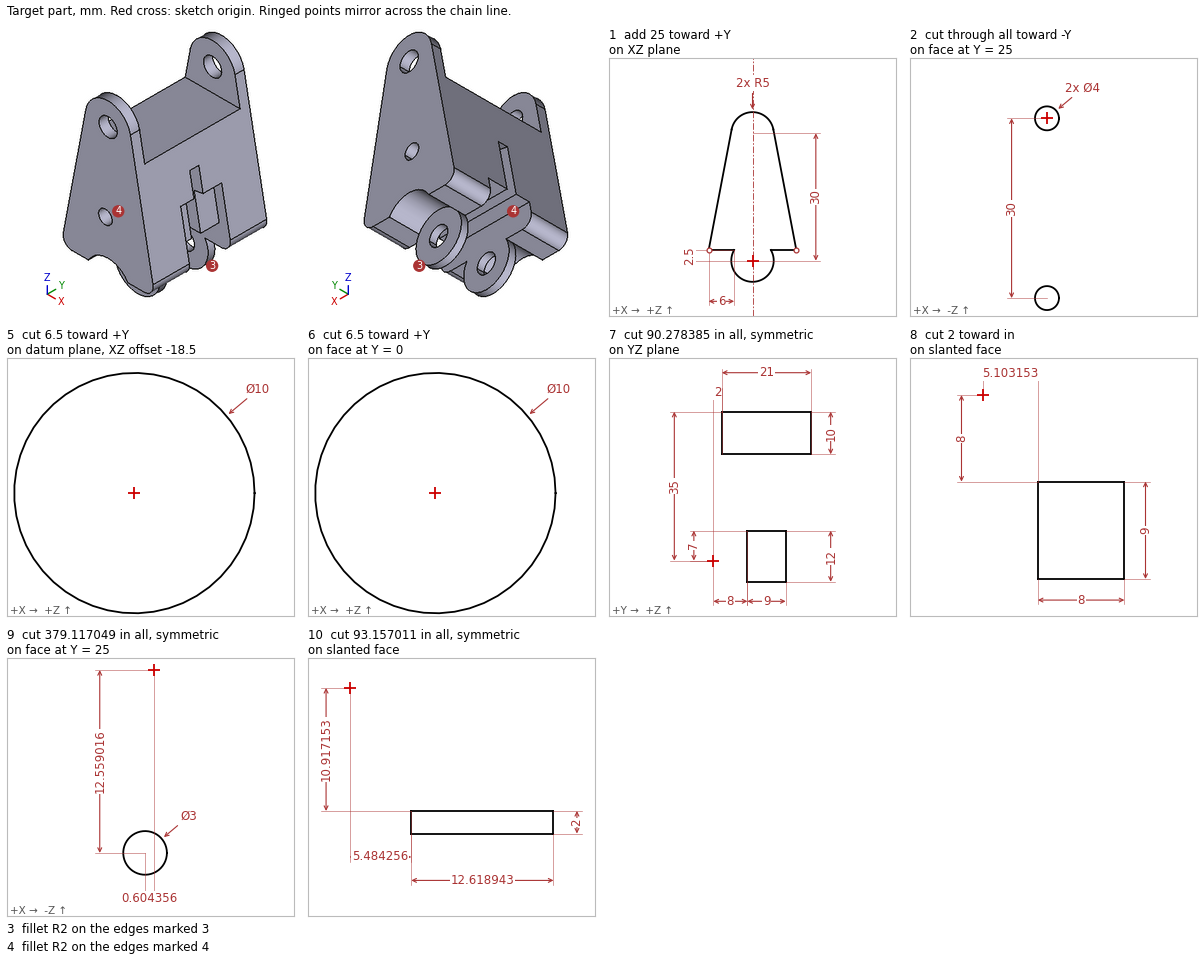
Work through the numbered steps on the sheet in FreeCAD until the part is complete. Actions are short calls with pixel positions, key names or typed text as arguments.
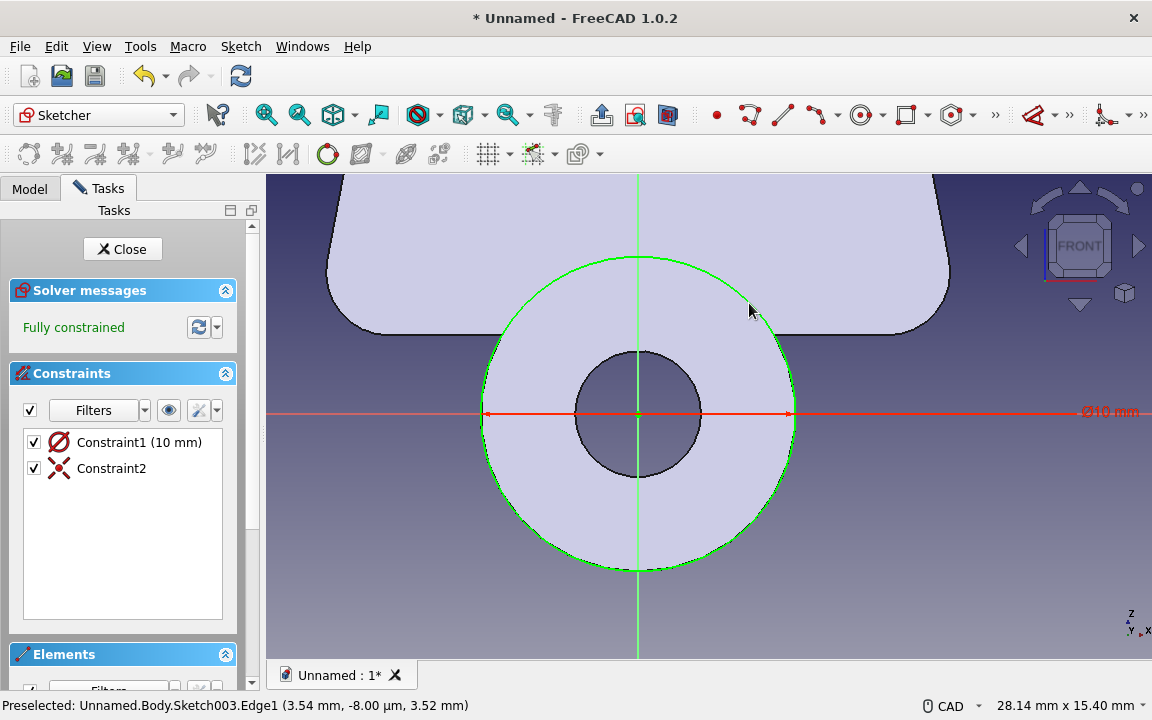
click(123, 249)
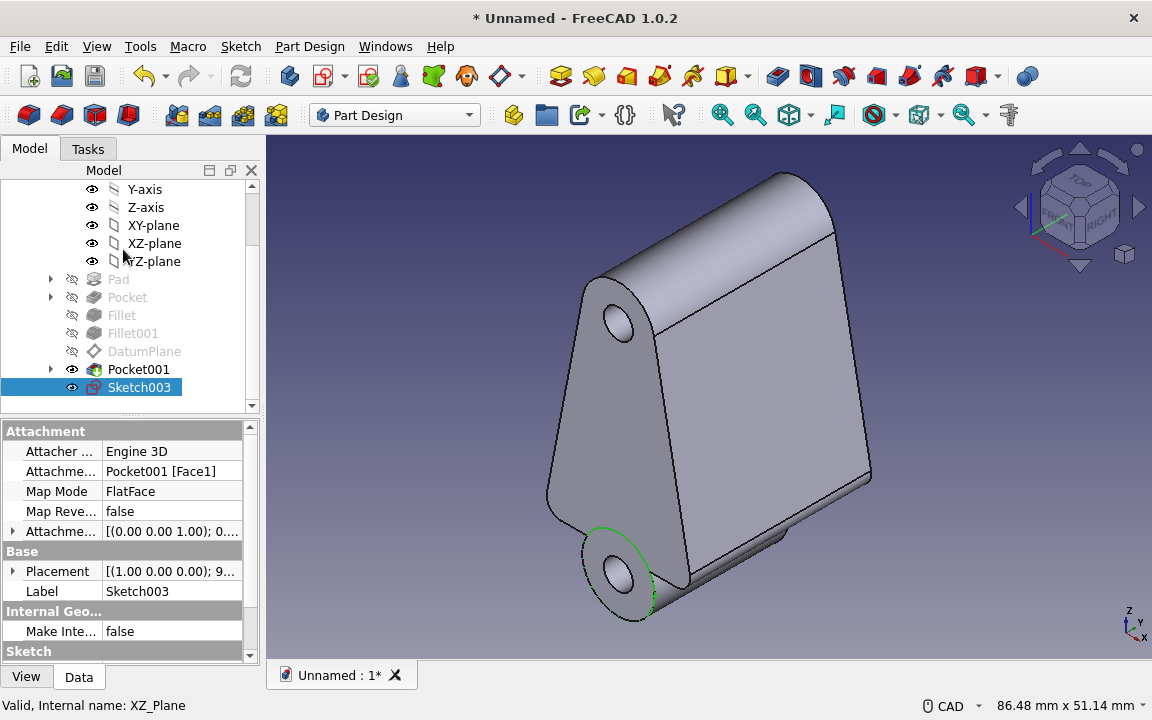
click(778, 76)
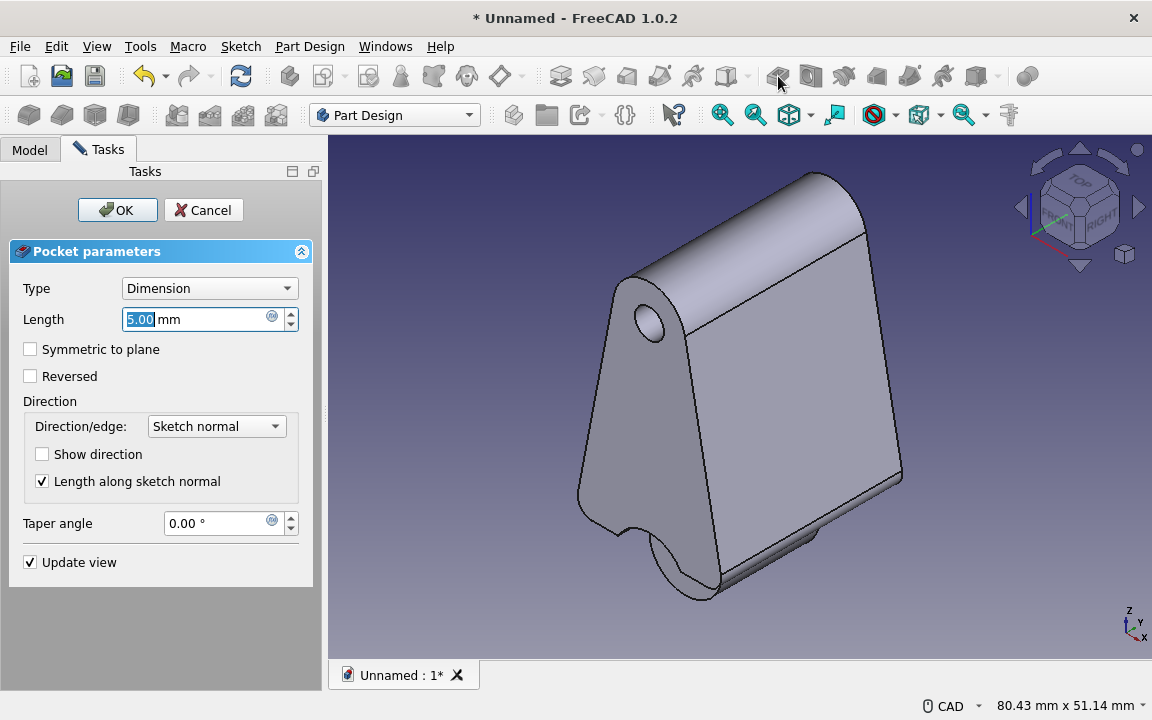
text(6.5)
key(Tab)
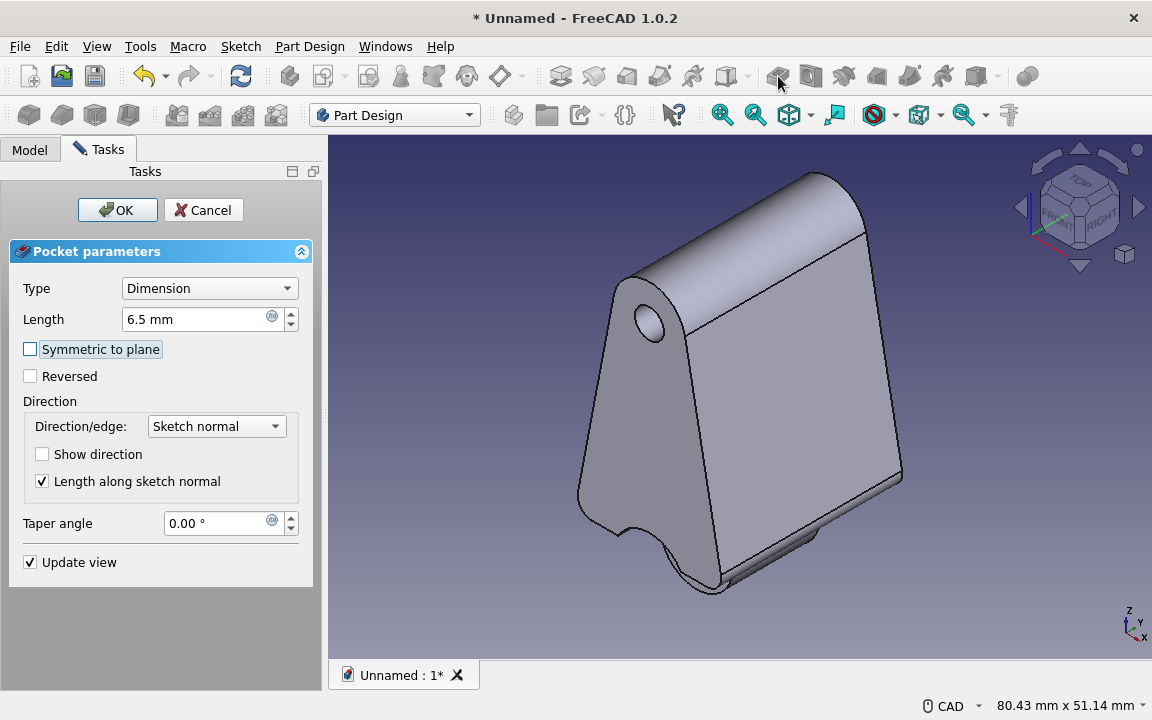
click(118, 210)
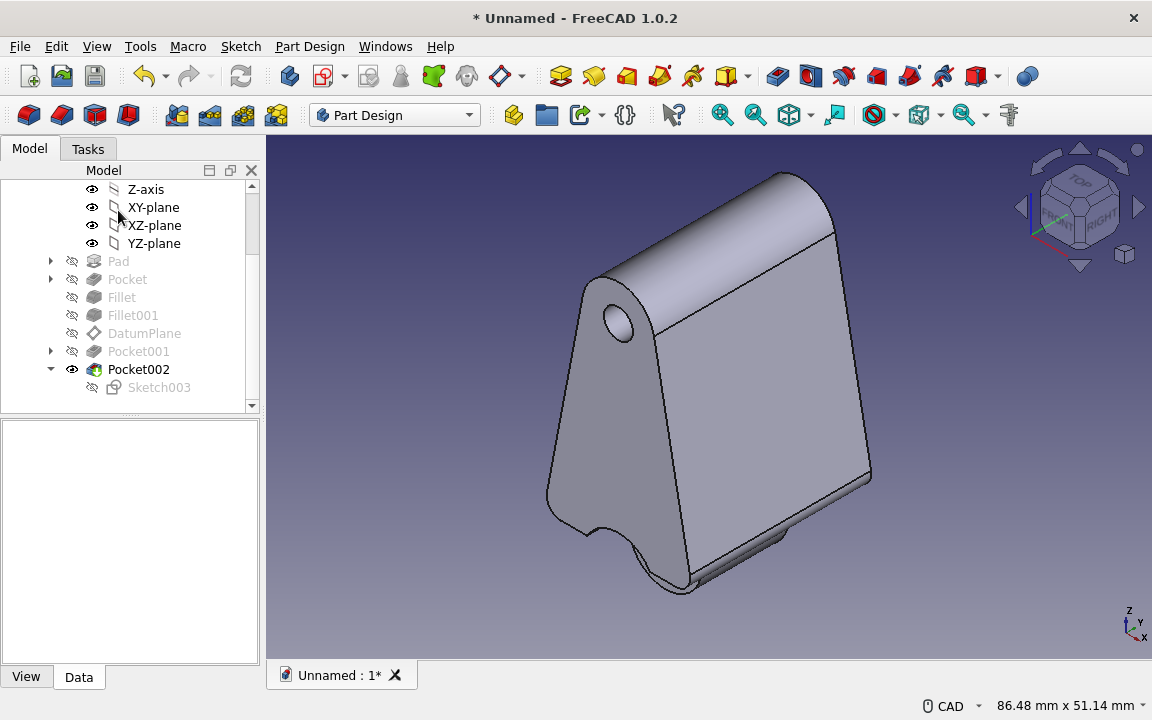
click(322, 76)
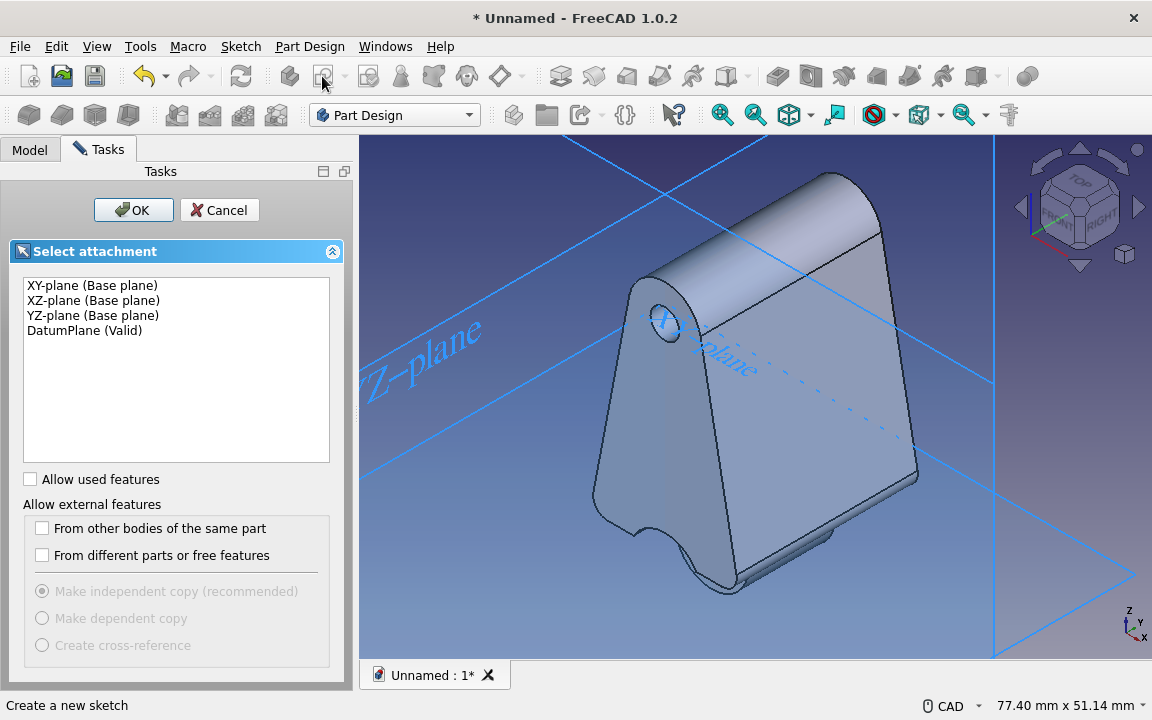
click(84, 316)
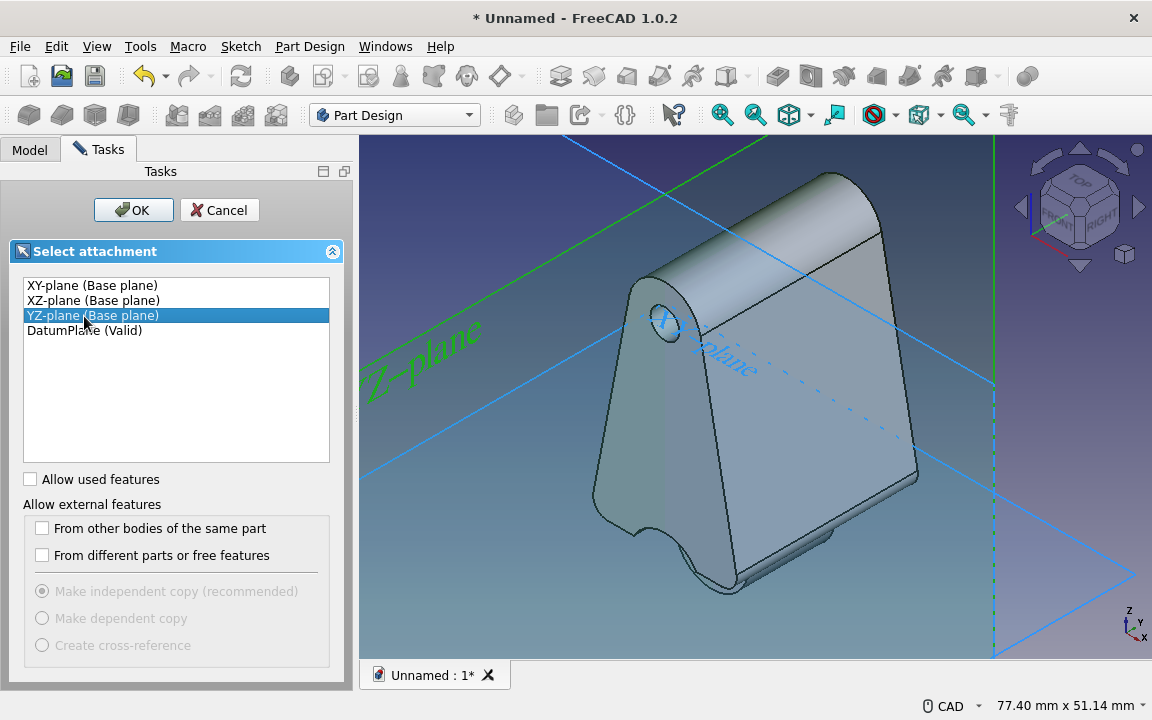
click(134, 210)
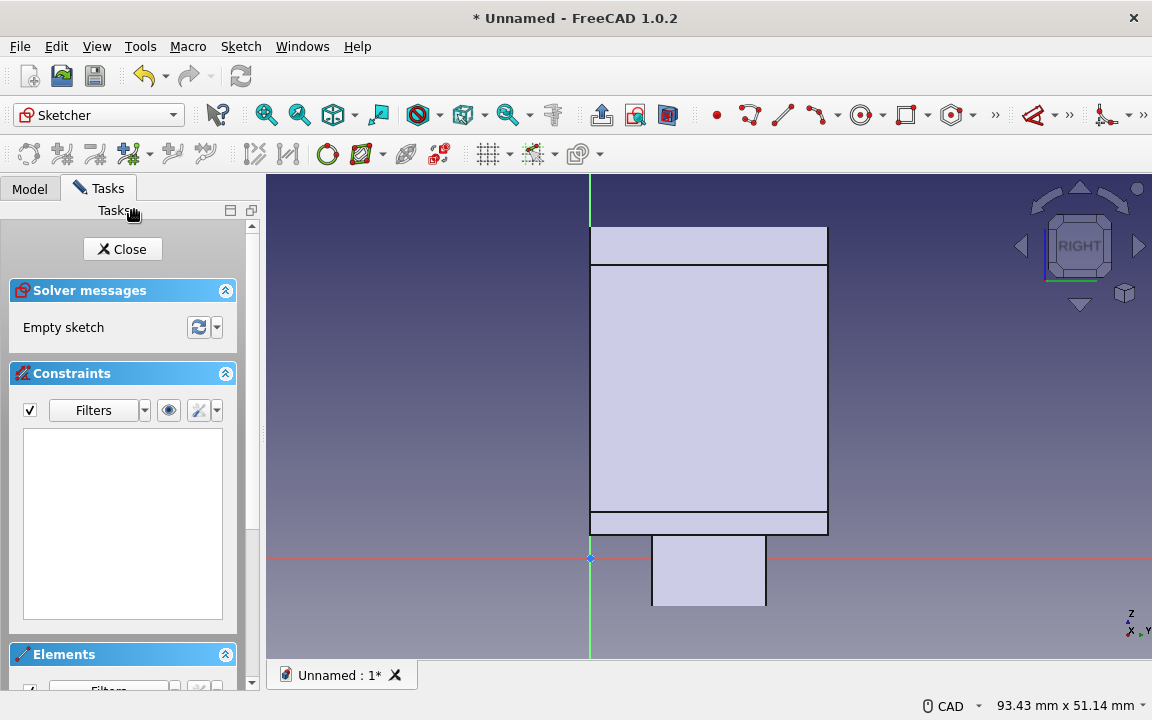
key(q)
key(s)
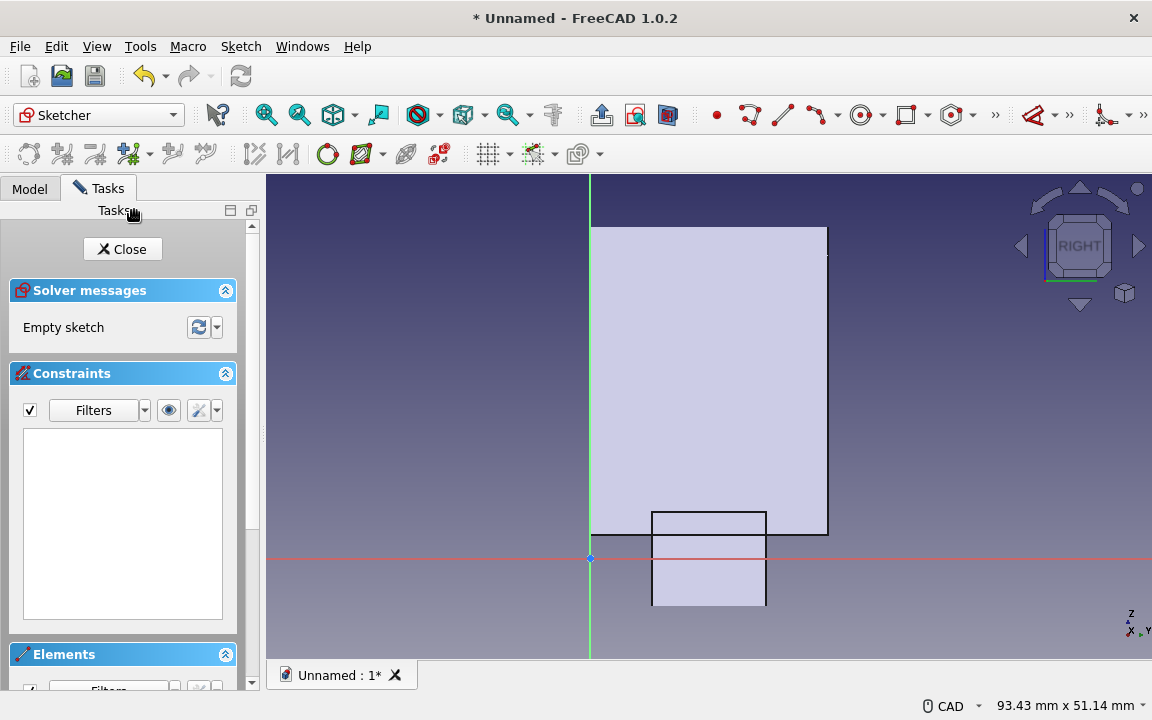
scroll(374, 417, down, 1)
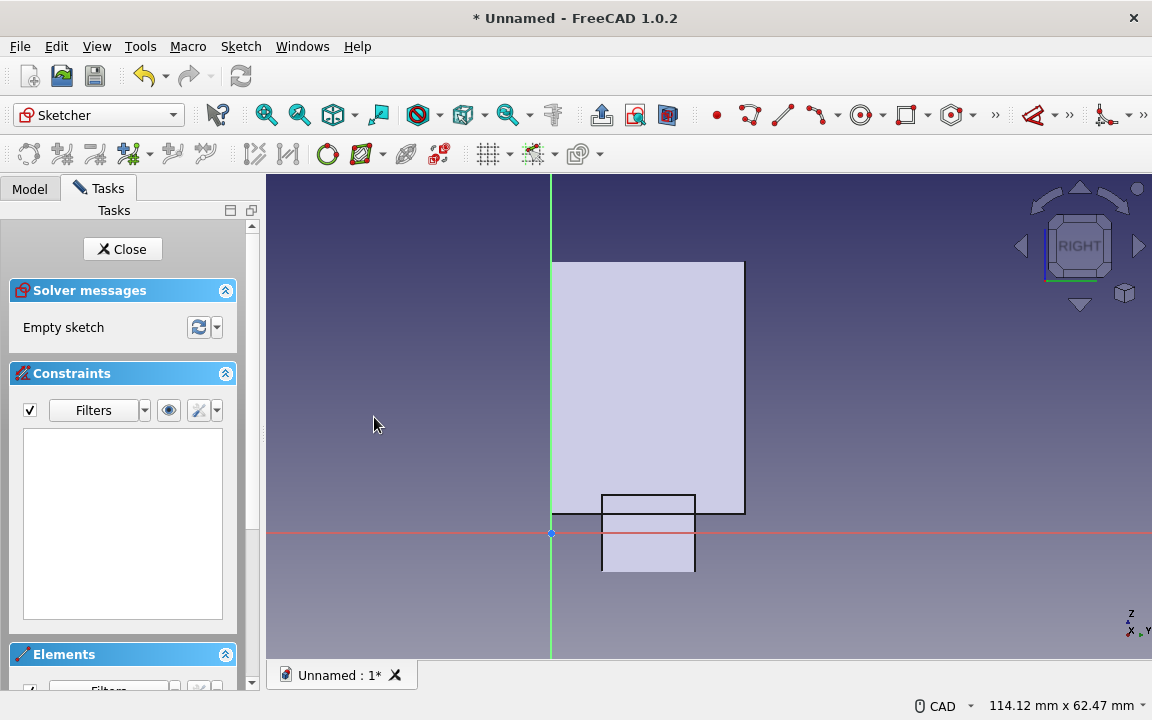
click(906, 116)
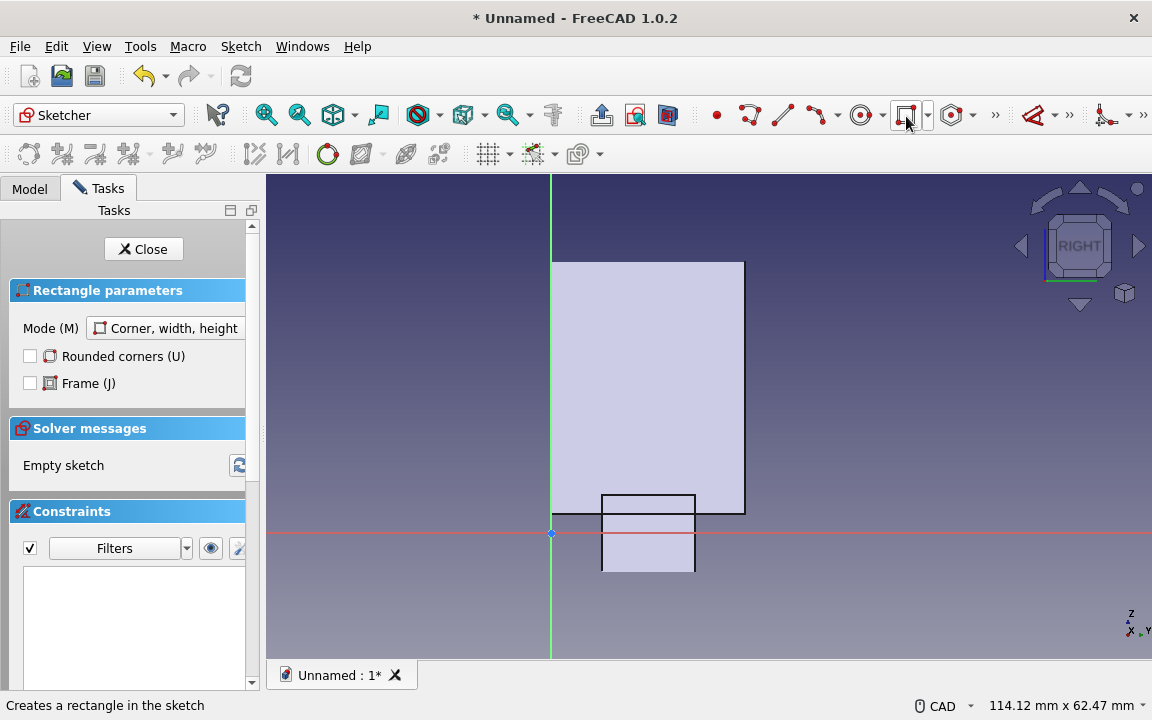
click(567, 261)
move(730, 339)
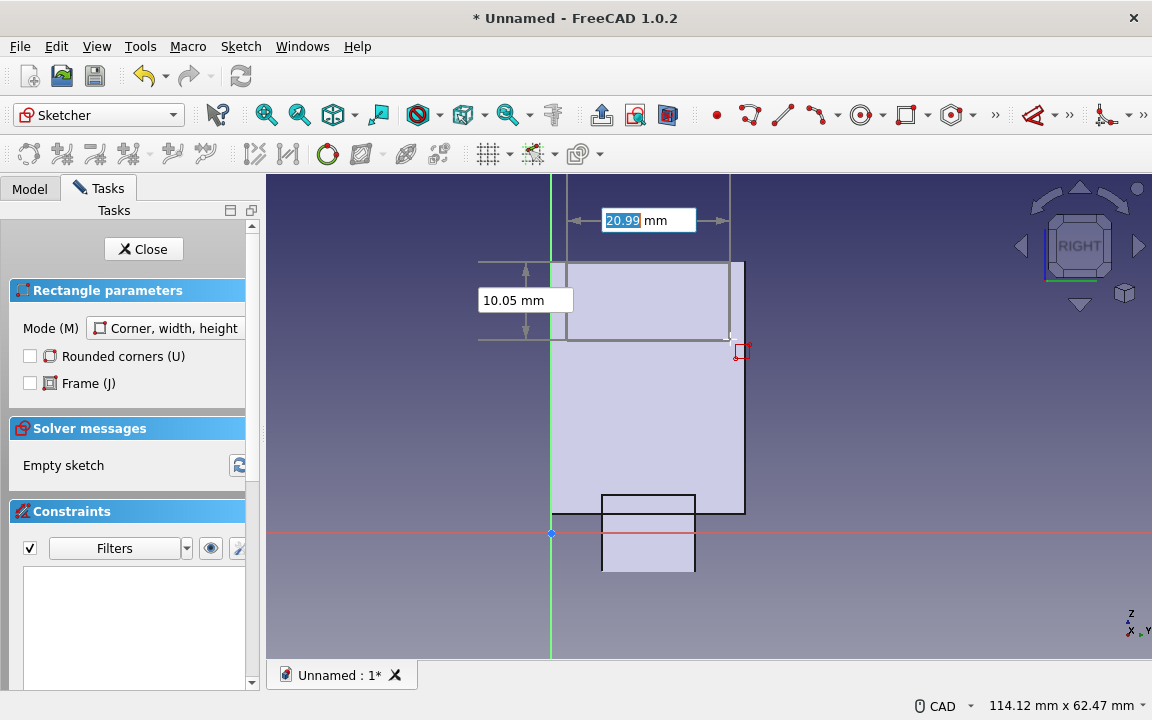
text(21)
key(Tab)
text(10)
key(Return)